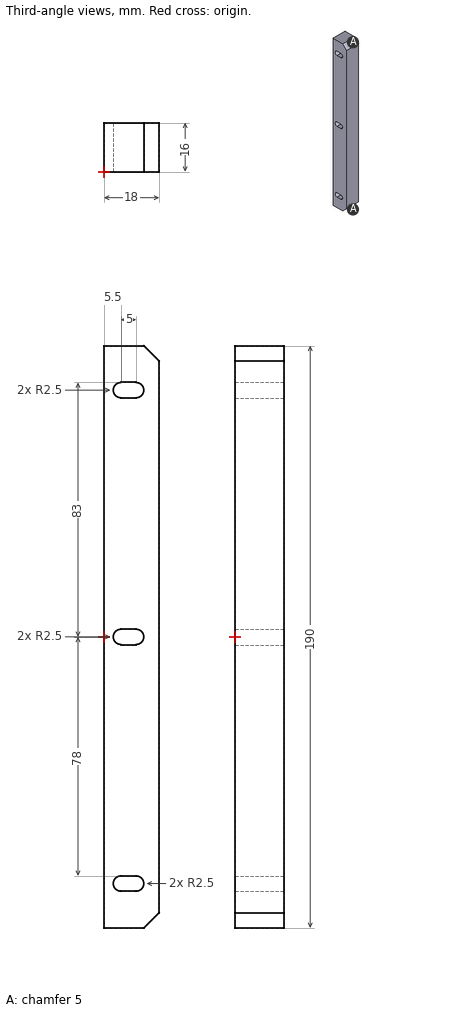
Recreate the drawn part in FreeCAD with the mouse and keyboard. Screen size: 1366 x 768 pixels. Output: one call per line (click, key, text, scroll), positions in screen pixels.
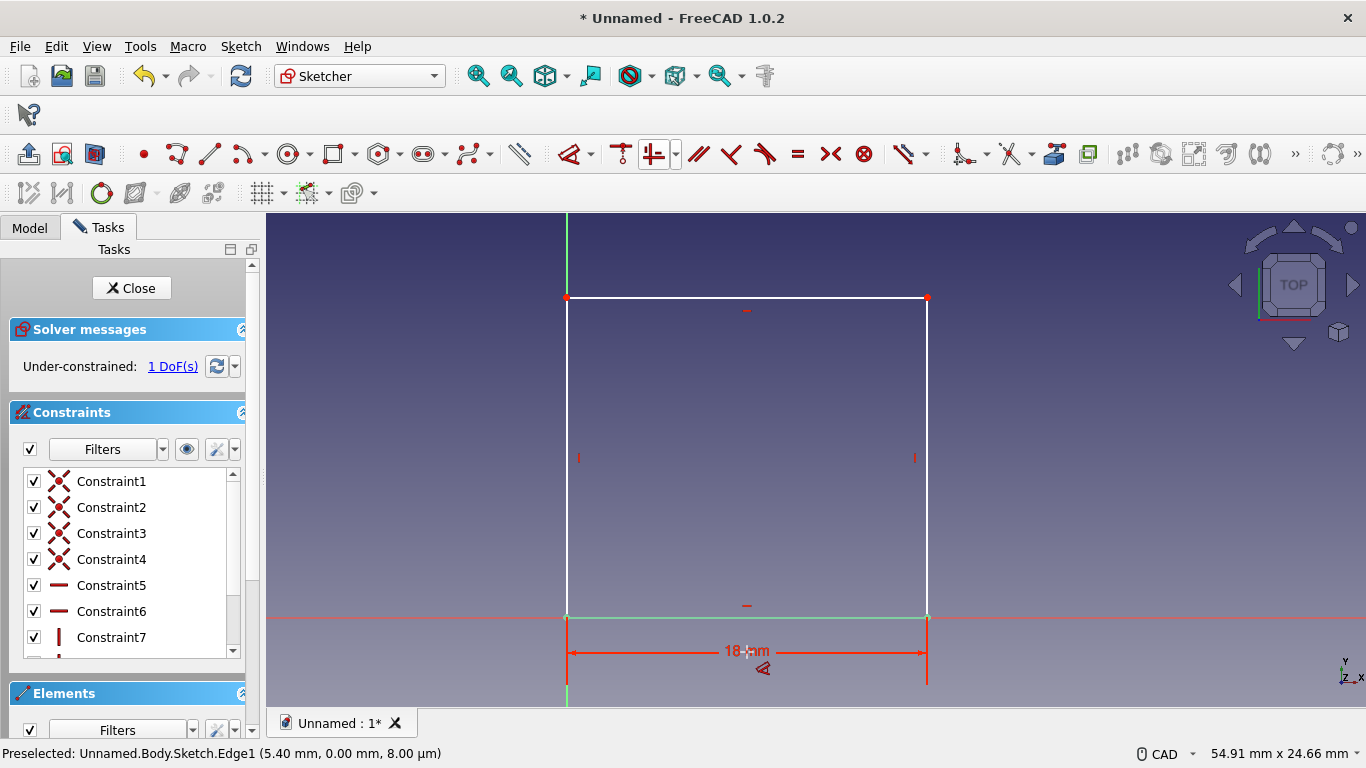
click(927, 522)
click(961, 458)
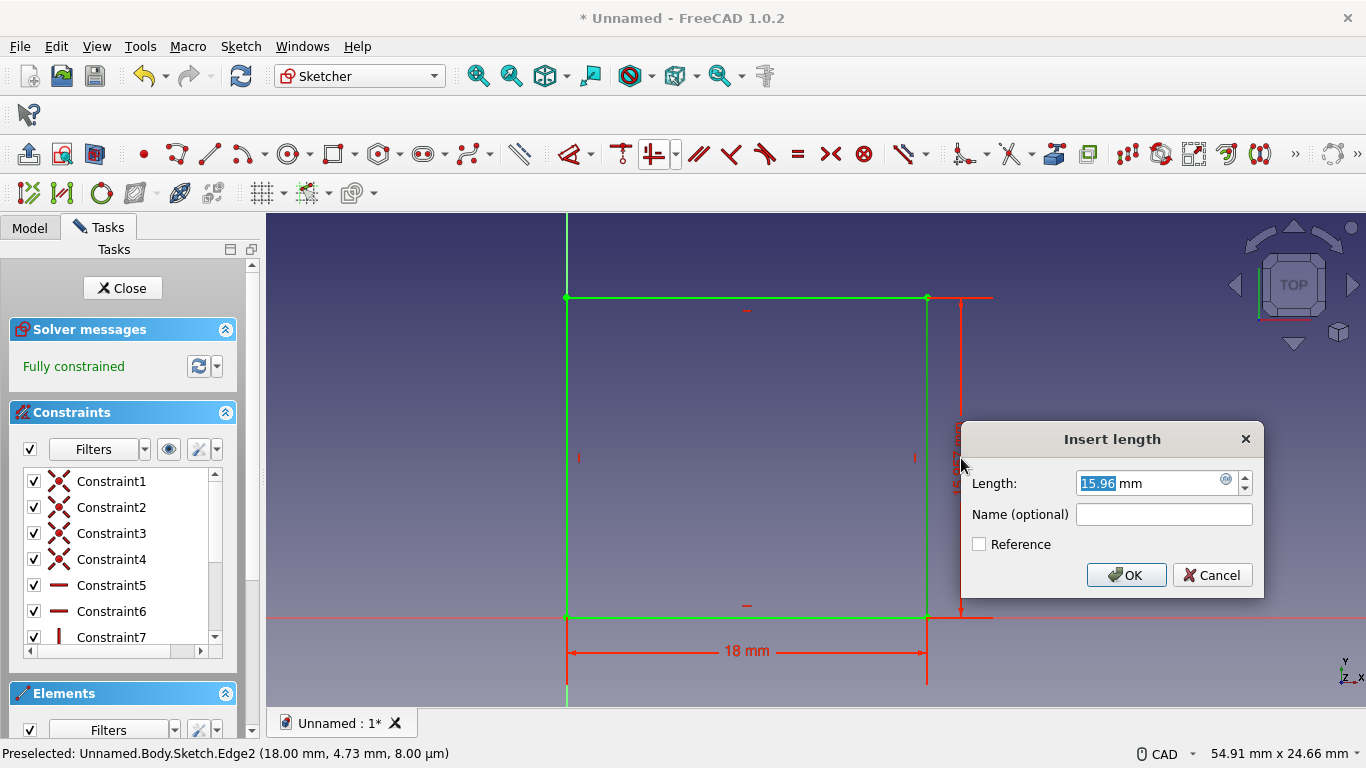
text(16)
key(Return)
key(Escape)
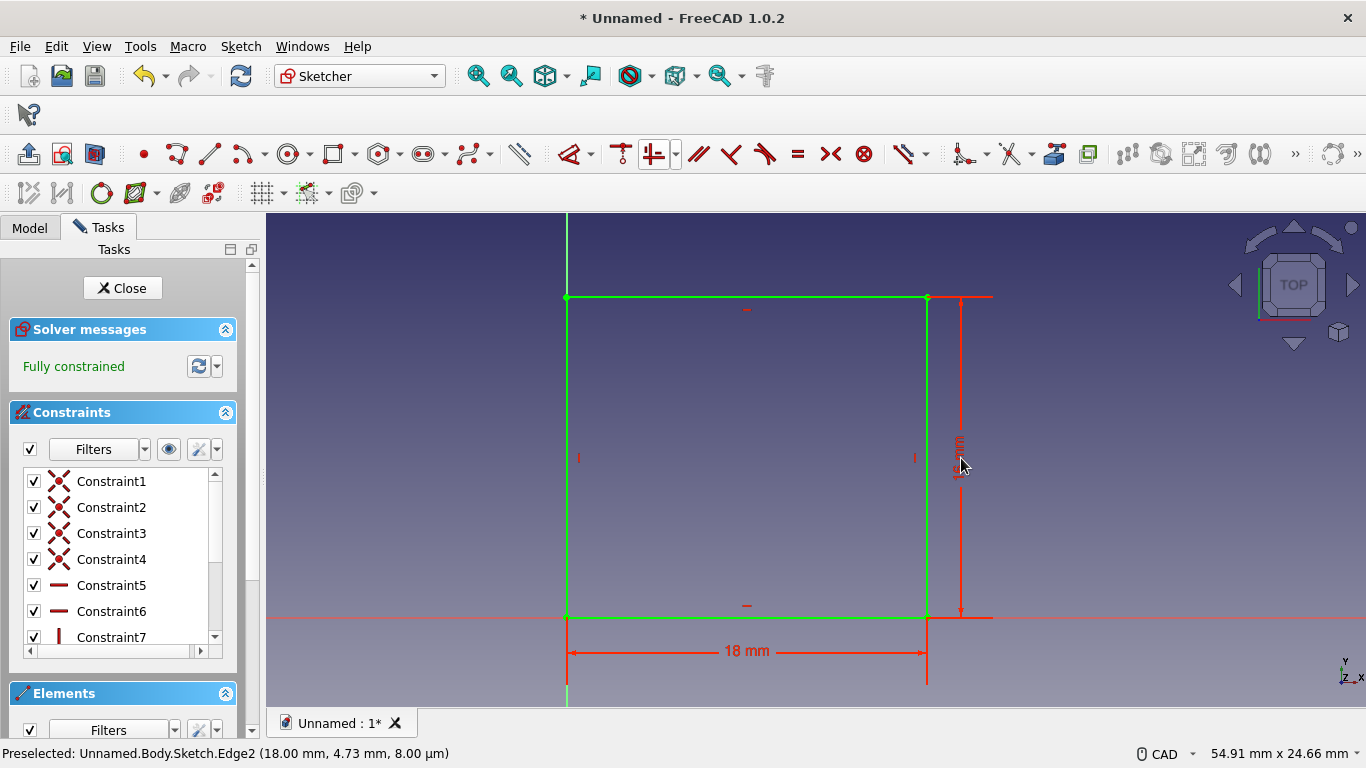
click(123, 288)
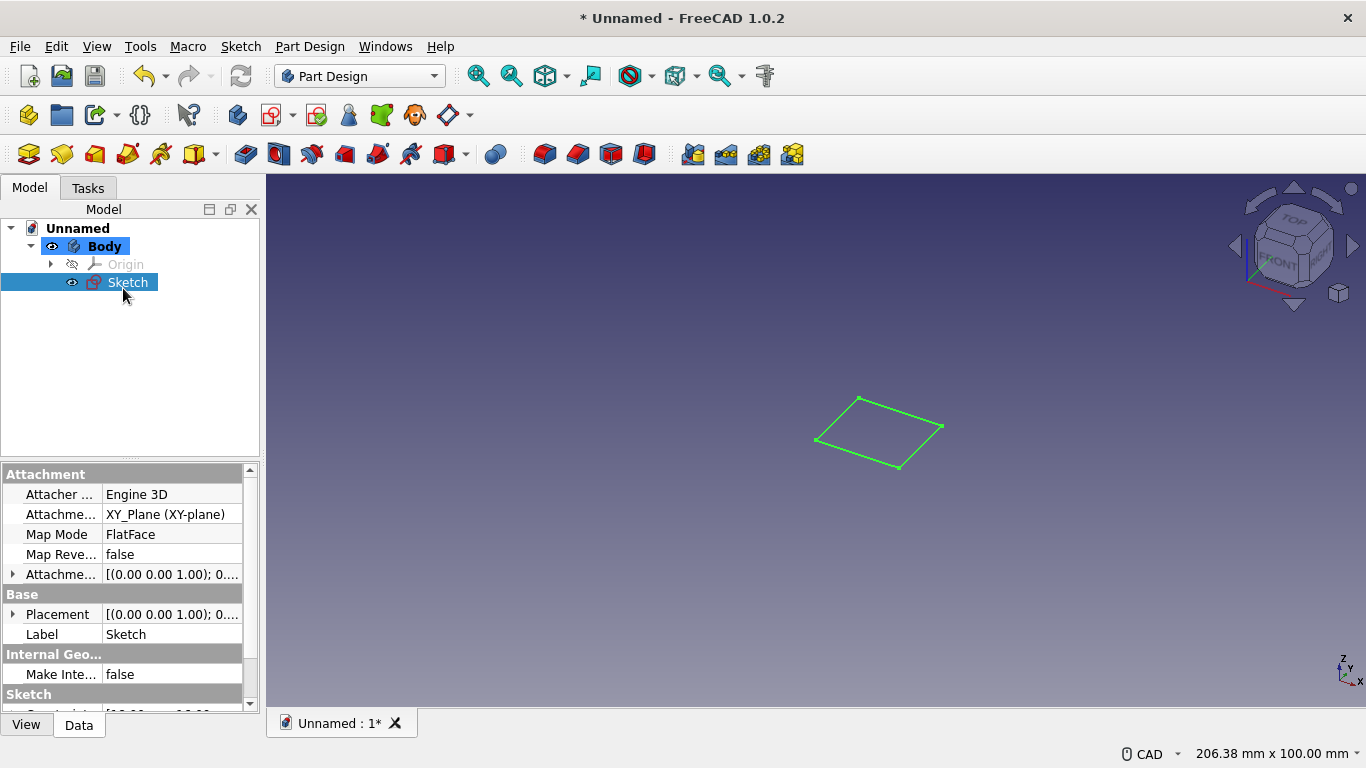
click(29, 154)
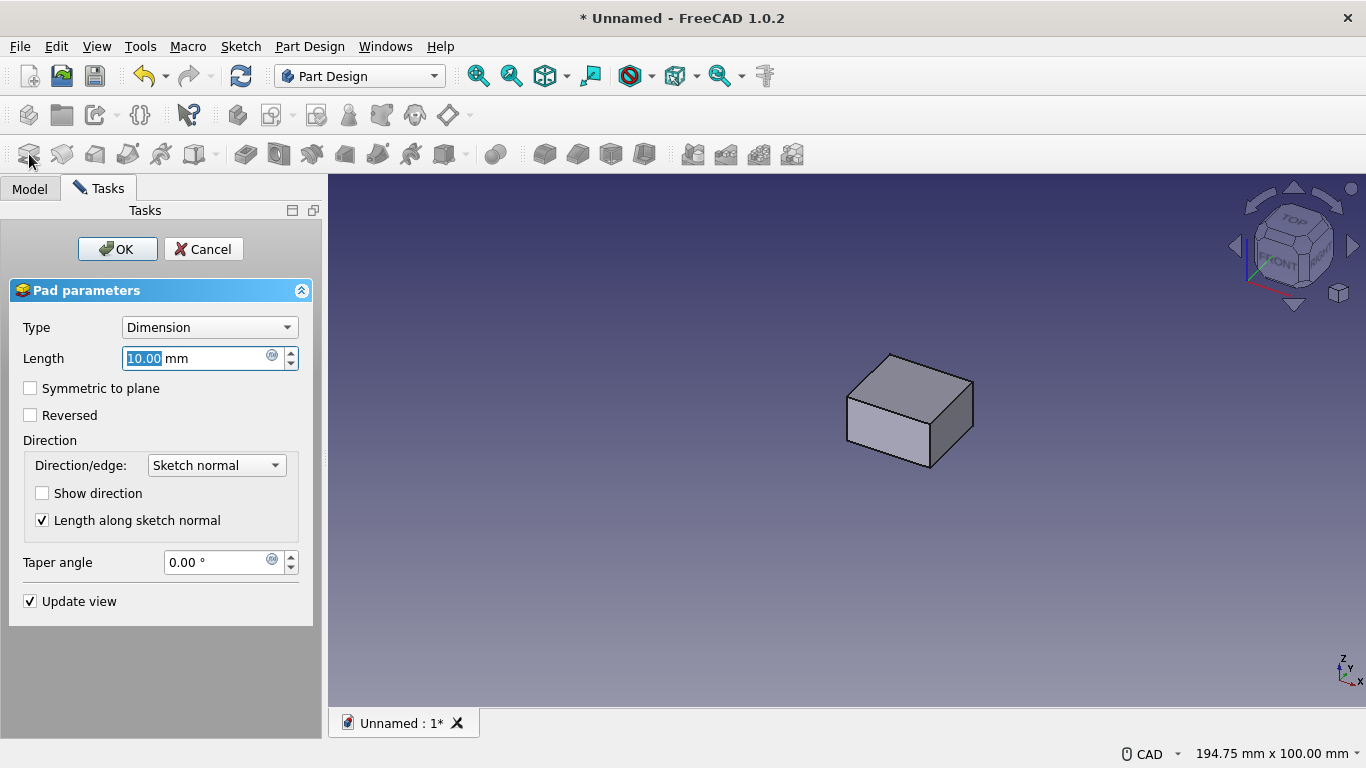
text(190)
key(Tab)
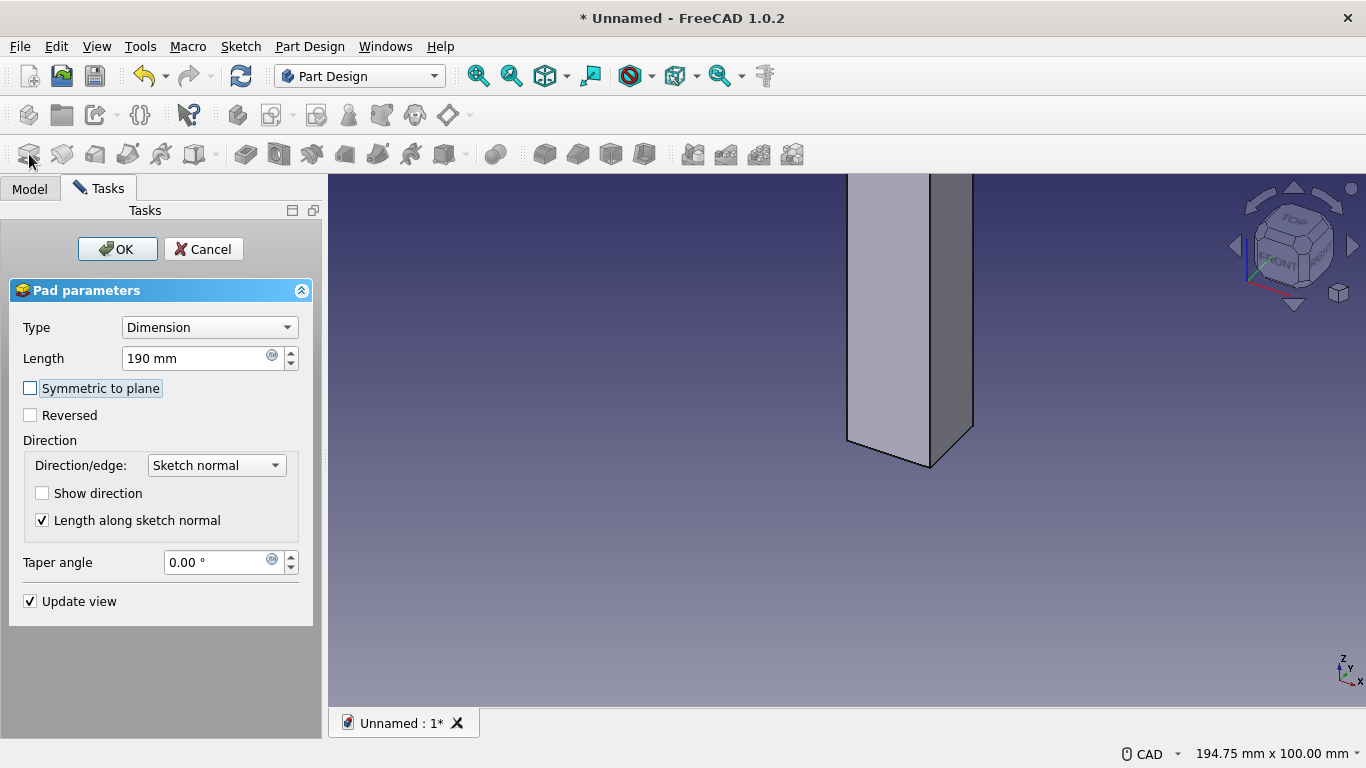
click(31, 388)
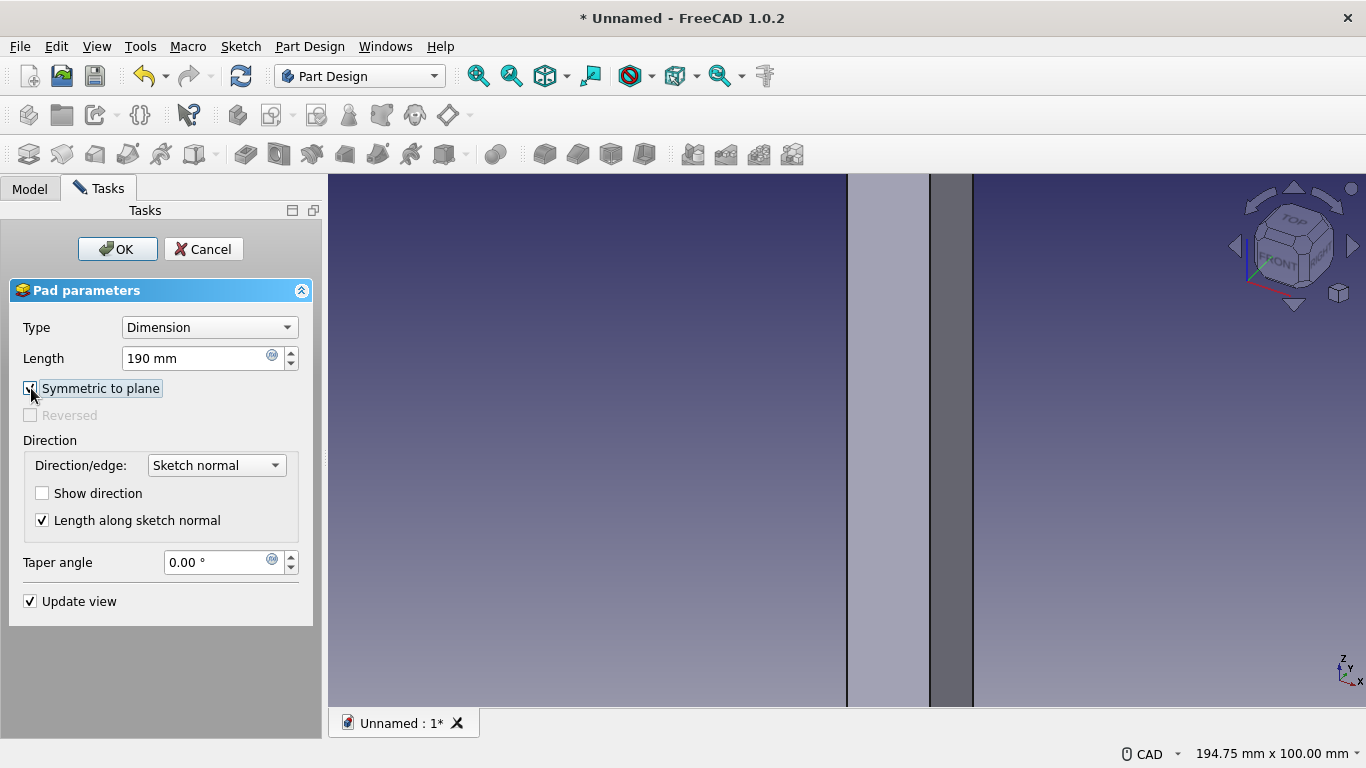
click(118, 249)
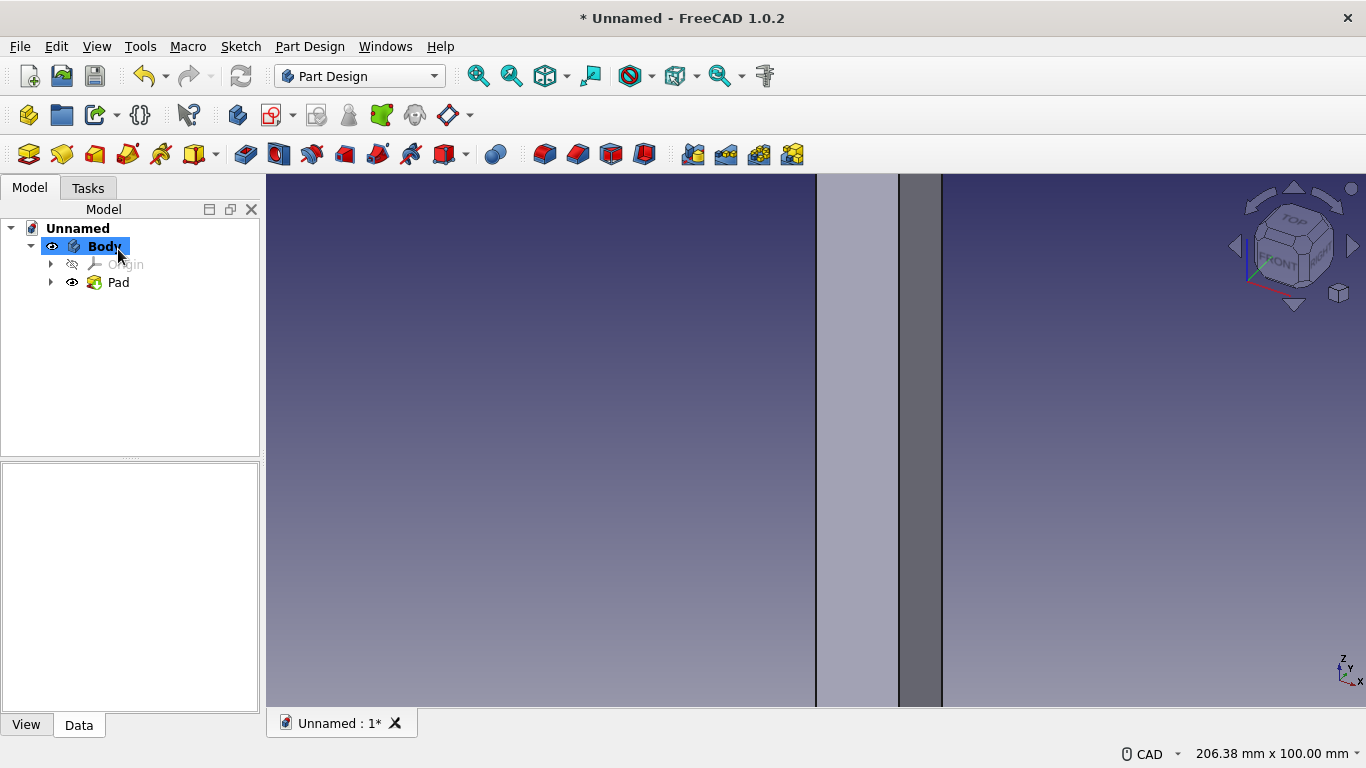
click(479, 76)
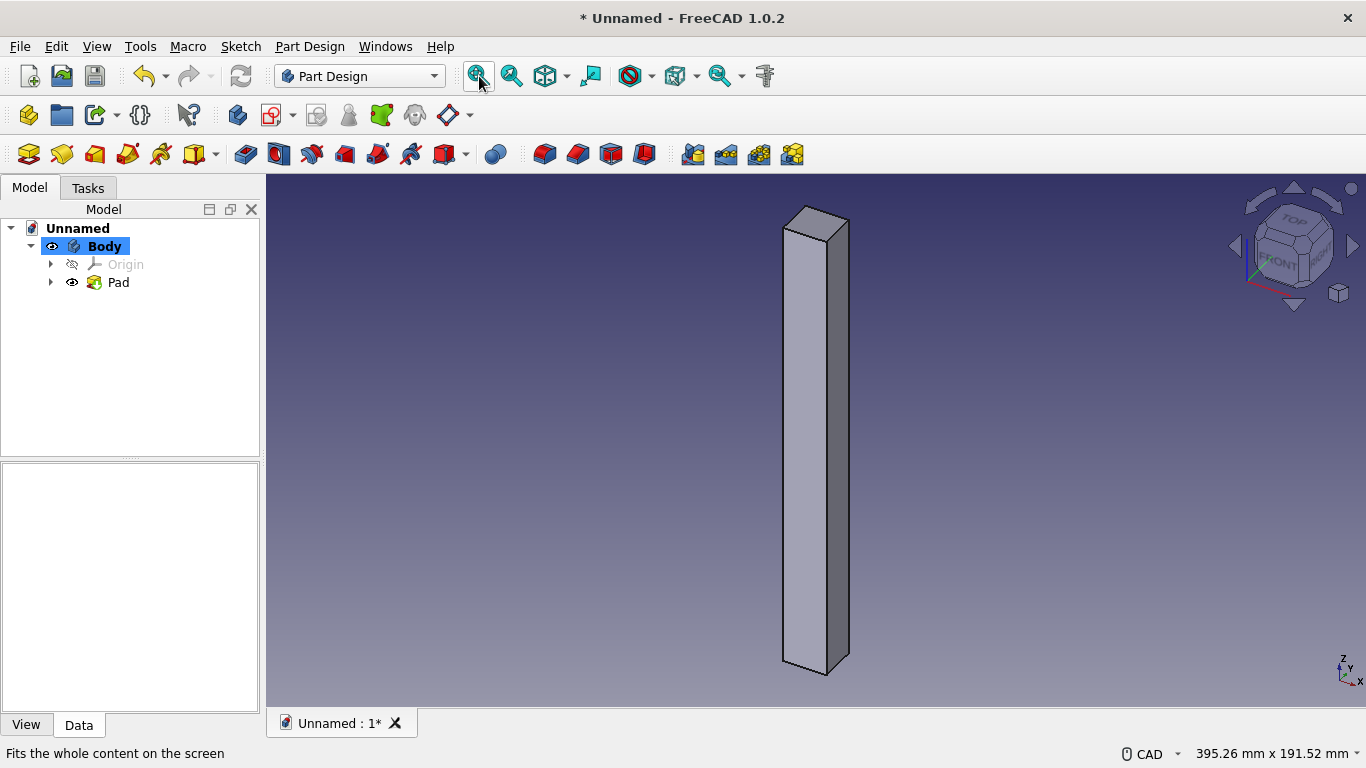
click(838, 230)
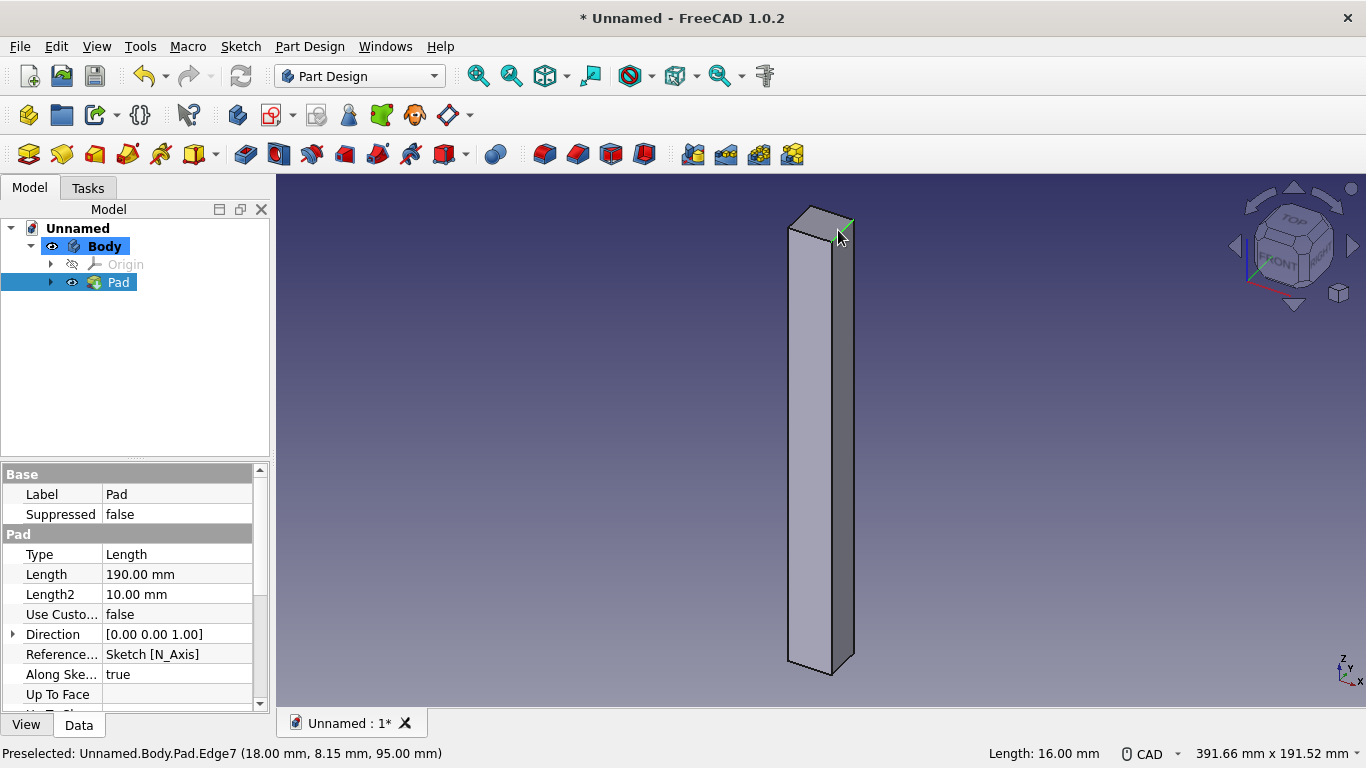
key(0)